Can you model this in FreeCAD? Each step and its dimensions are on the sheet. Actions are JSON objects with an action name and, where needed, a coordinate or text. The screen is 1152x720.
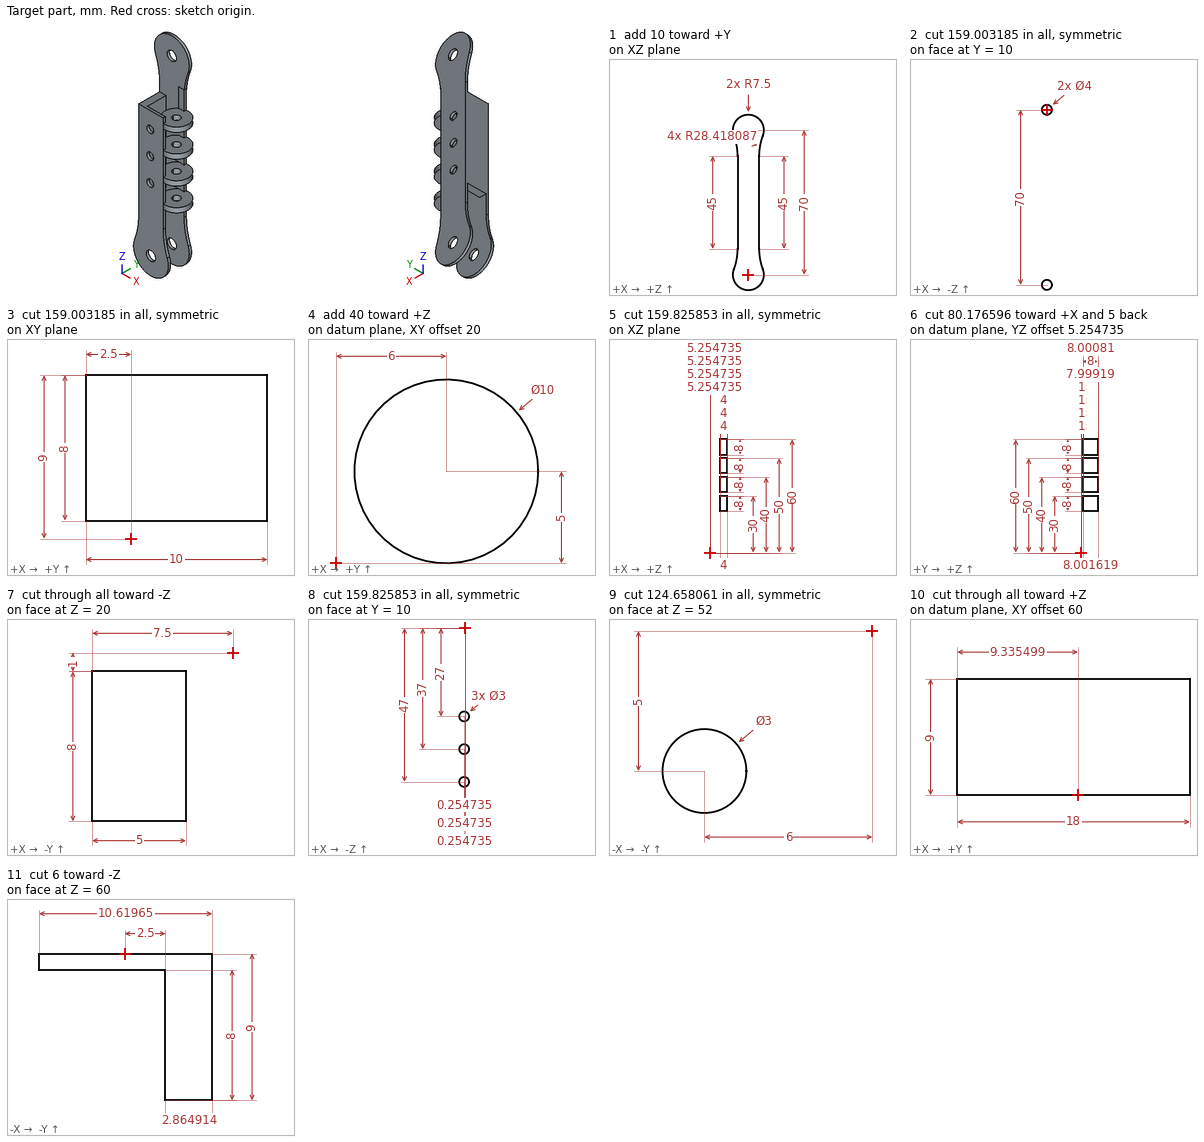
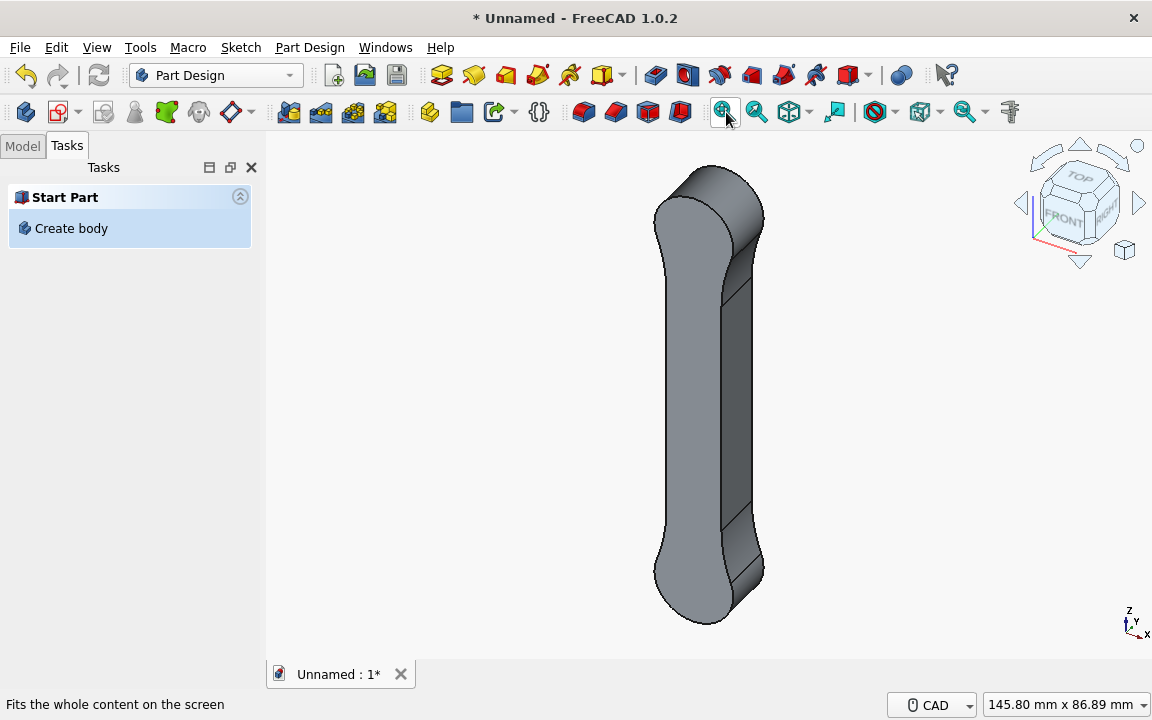
{"action": "key", "text": "4"}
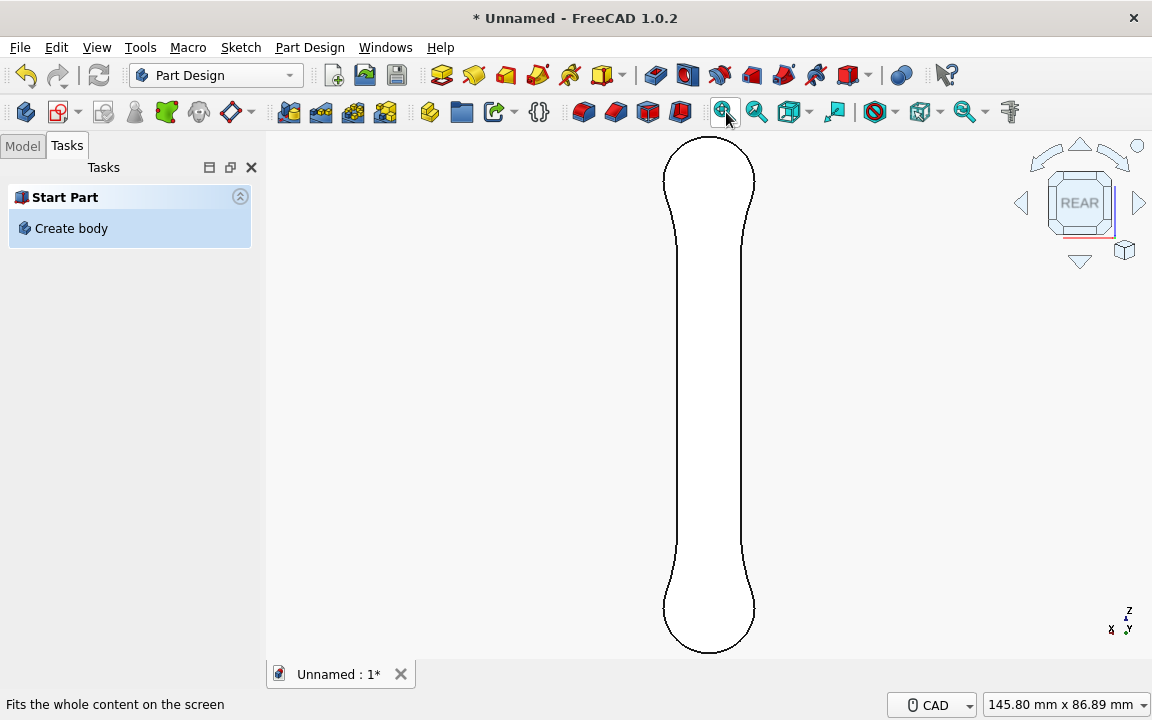
{"action": "left_click", "coordinate": [709, 615]}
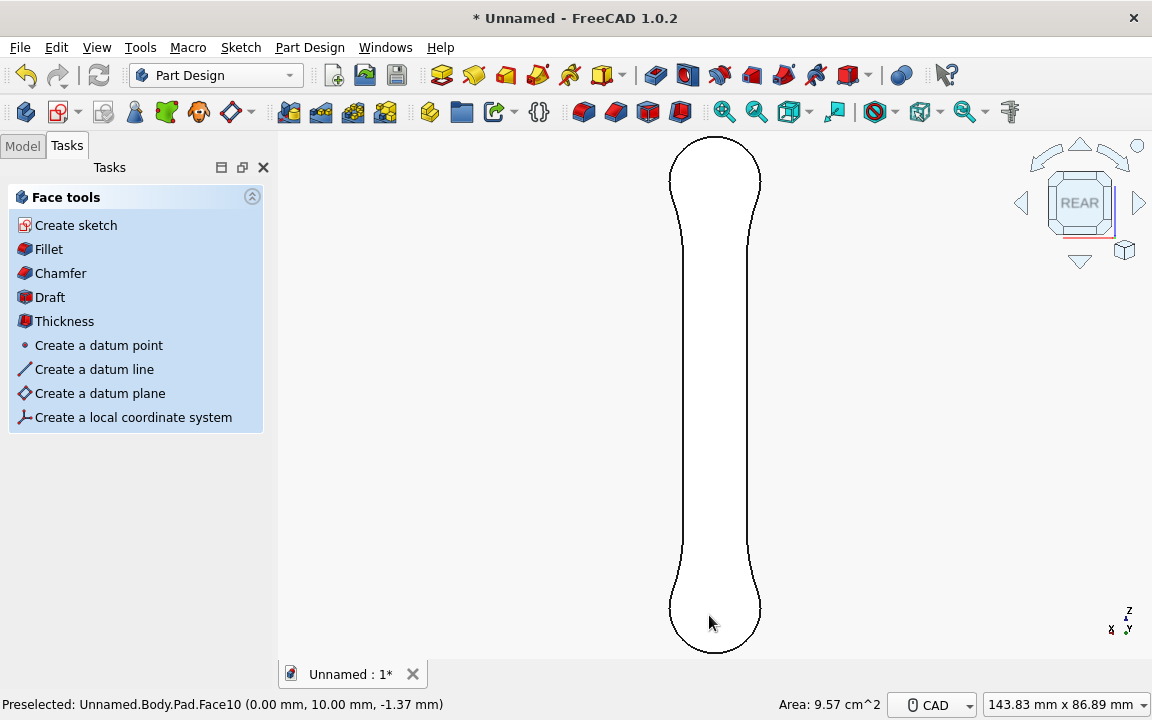
{"action": "left_click", "coordinate": [58, 112]}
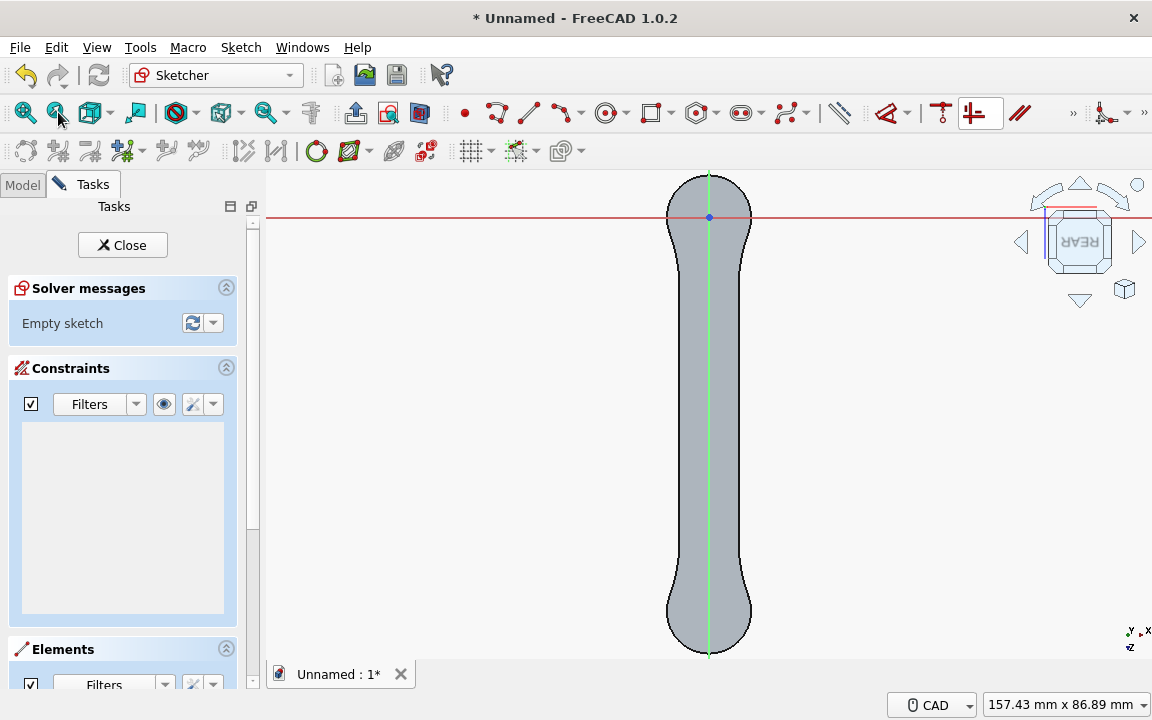
{"action": "scroll", "coordinate": [501, 415], "scroll_direction": "down", "scroll_amount": 2}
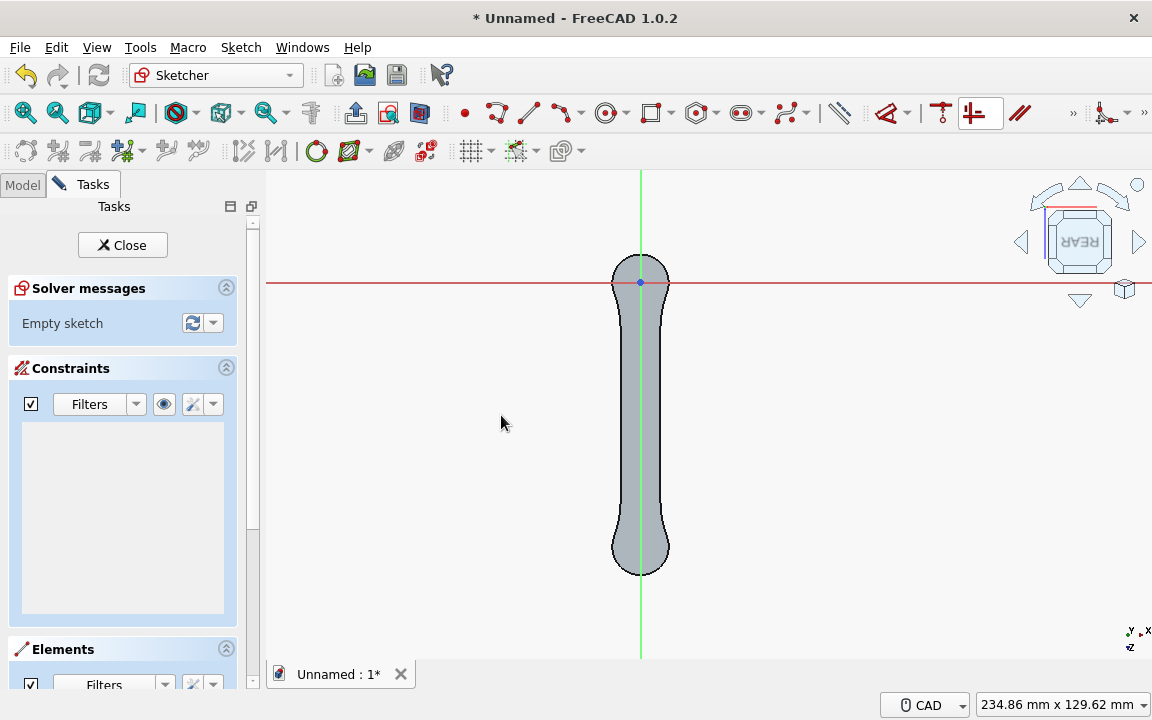
{"action": "left_click", "coordinate": [606, 114]}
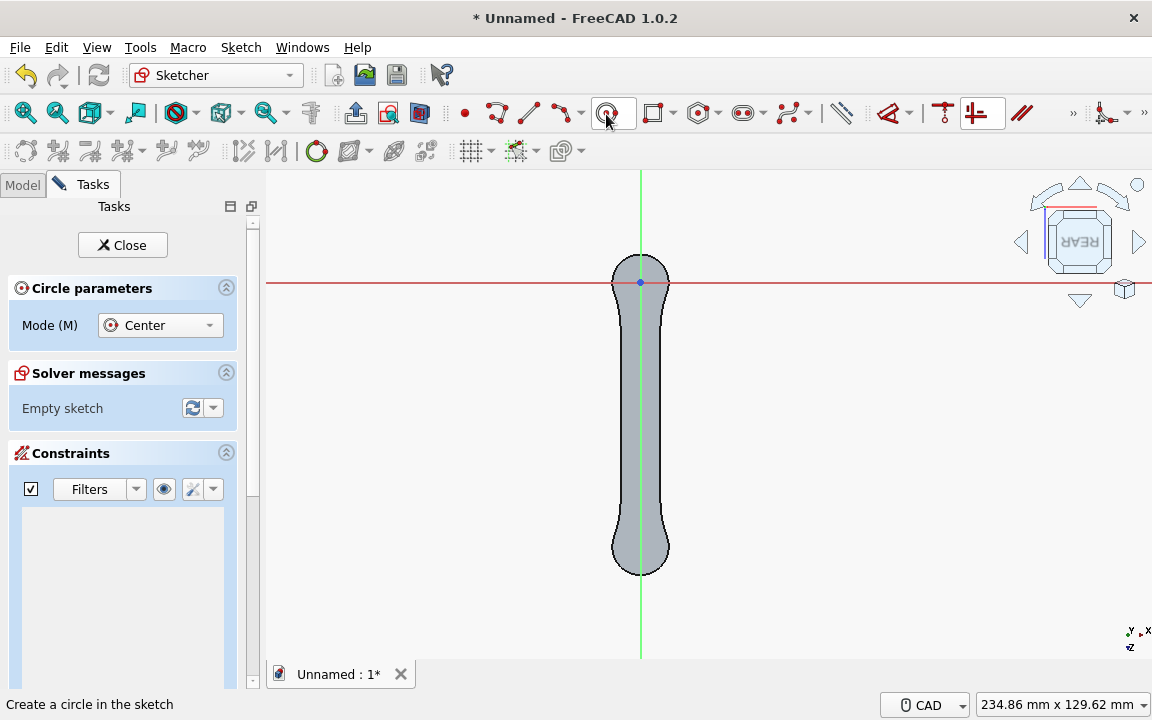
{"action": "scroll", "coordinate": [641, 283], "scroll_direction": "up", "scroll_amount": 6}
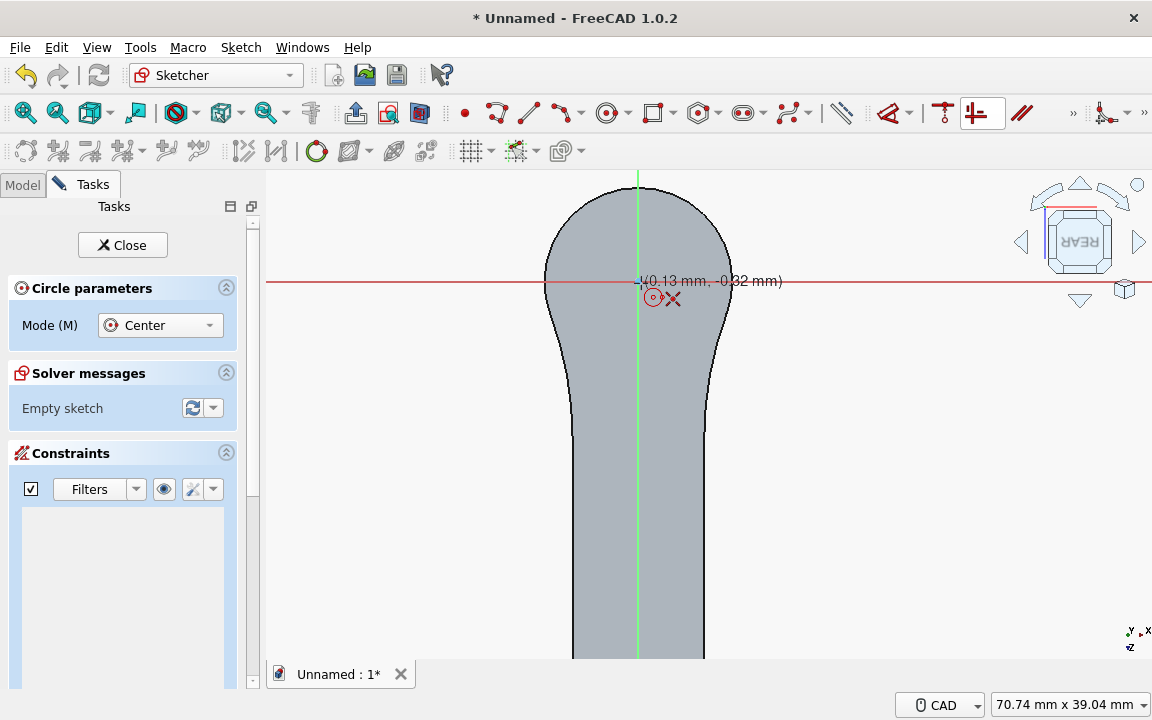
{"action": "left_click", "coordinate": [638, 282]}
{"action": "left_click", "coordinate": [656, 264]}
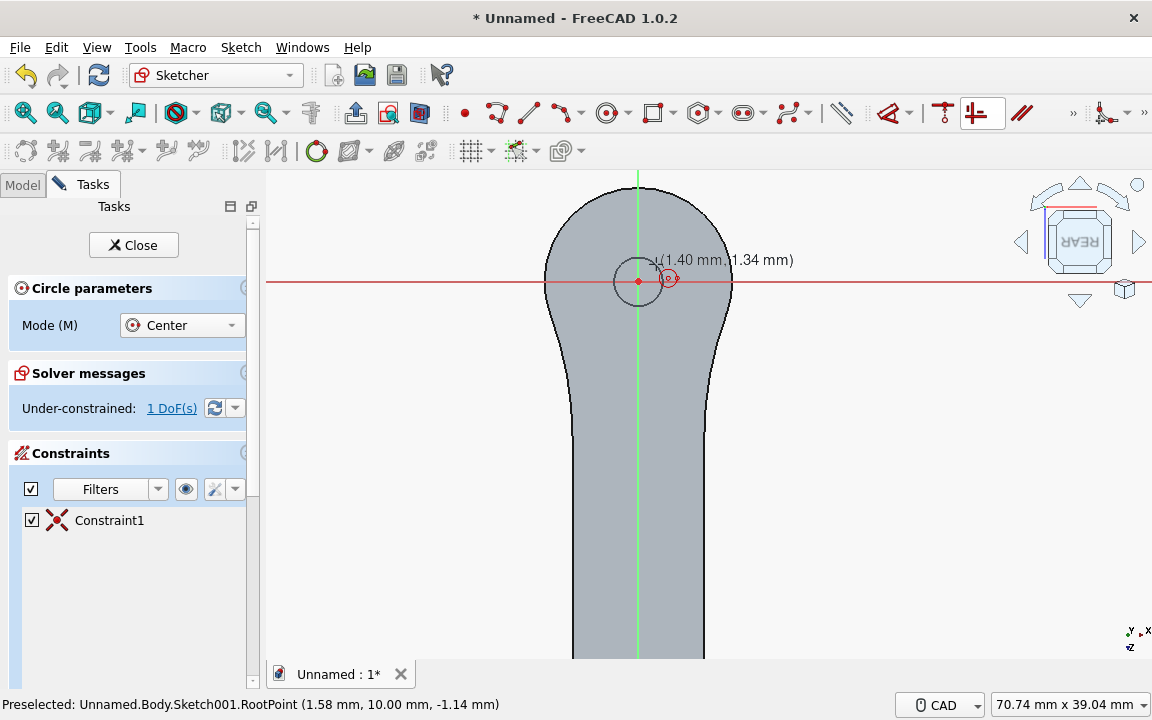
{"action": "scroll", "coordinate": [641, 283], "scroll_direction": "down", "scroll_amount": 6}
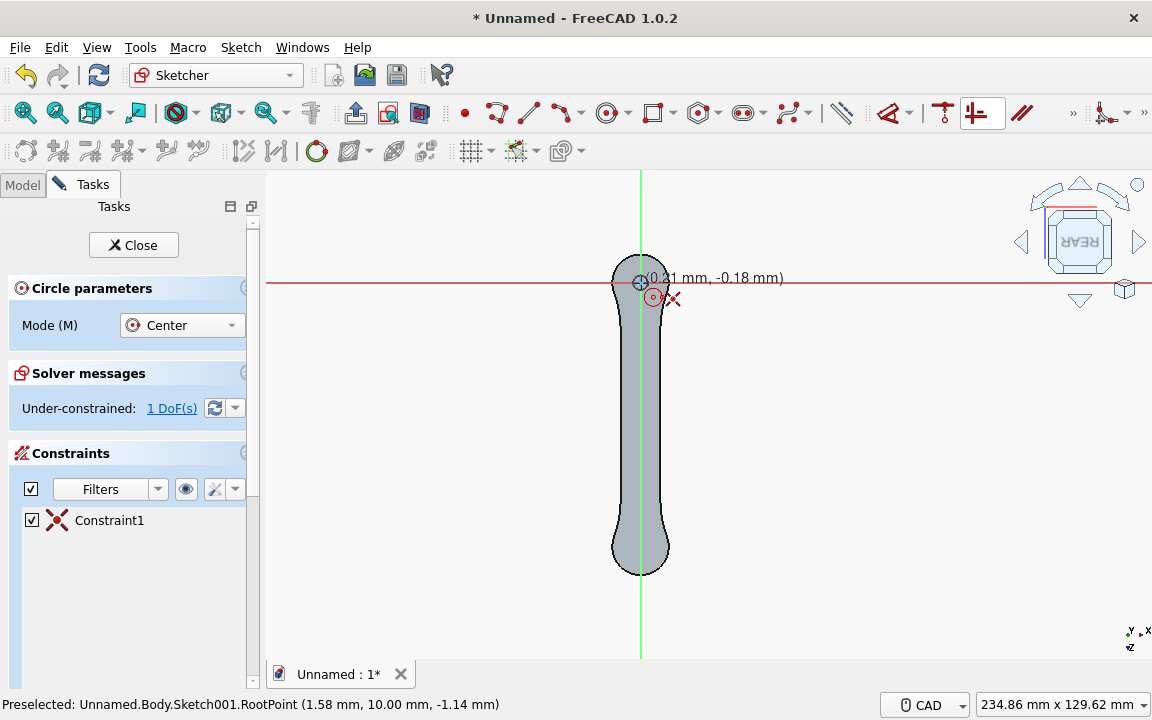
{"action": "scroll", "coordinate": [641, 547], "scroll_direction": "up", "scroll_amount": 6}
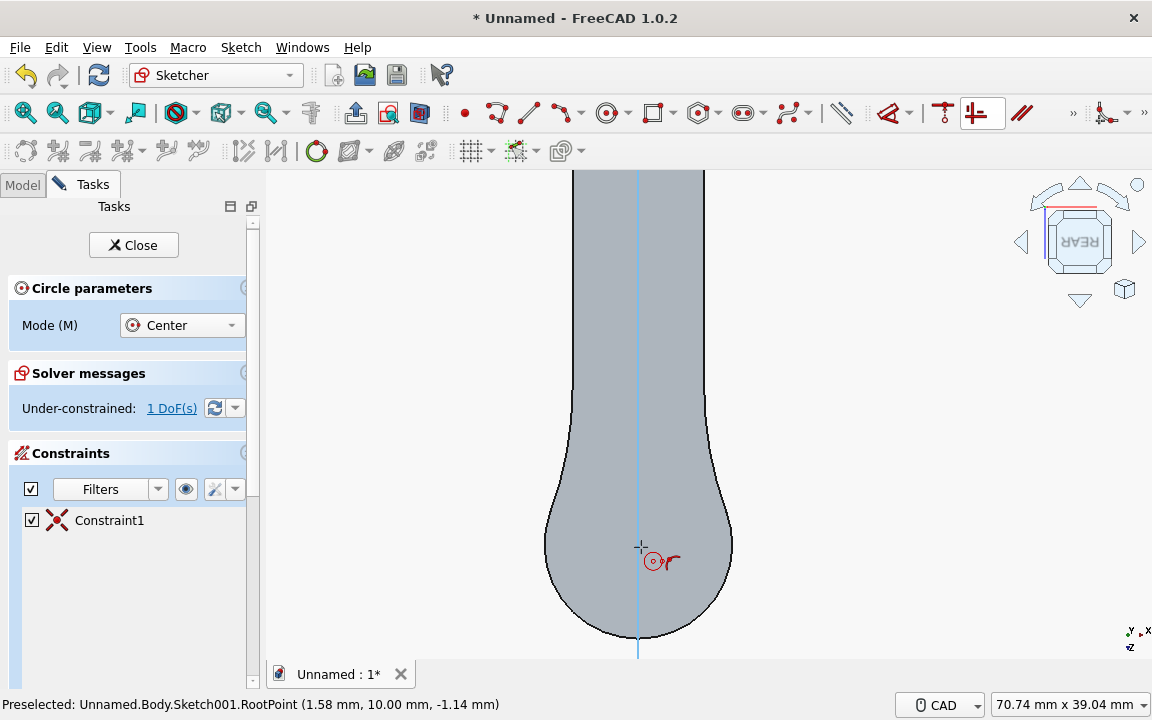
{"action": "left_click", "coordinate": [638, 545]}
{"action": "left_click", "coordinate": [656, 527]}
{"action": "key", "text": "Escape"}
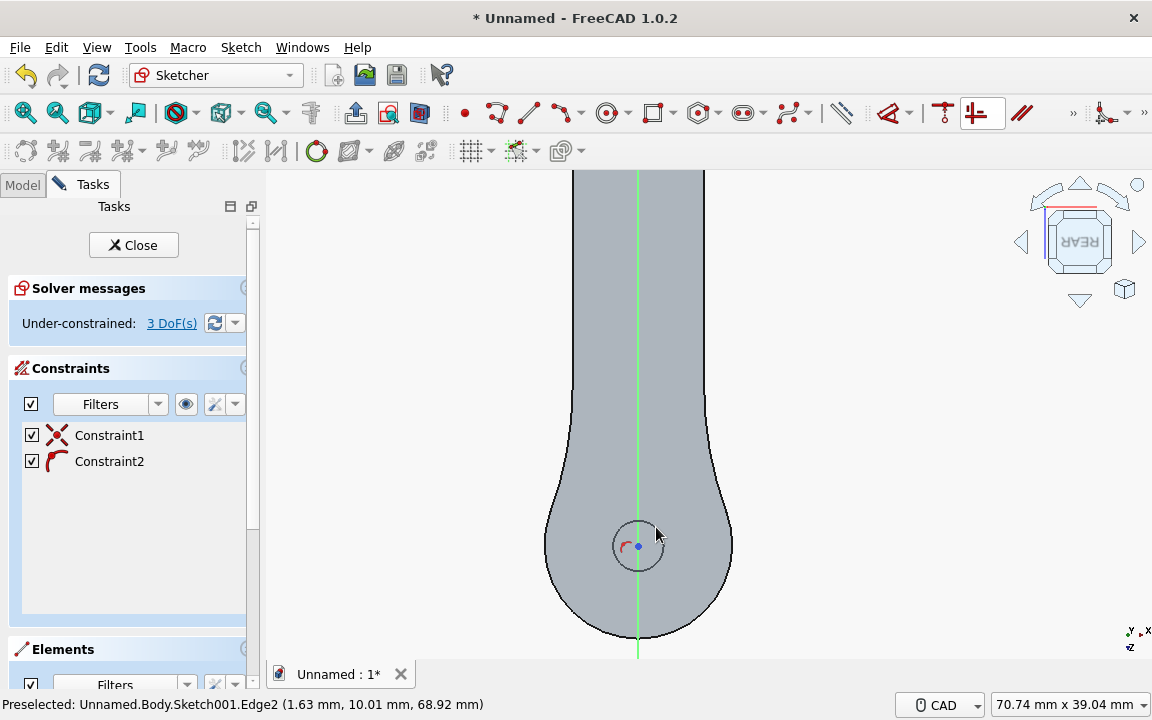
{"action": "scroll", "coordinate": [641, 547], "scroll_direction": "down", "scroll_amount": 6}